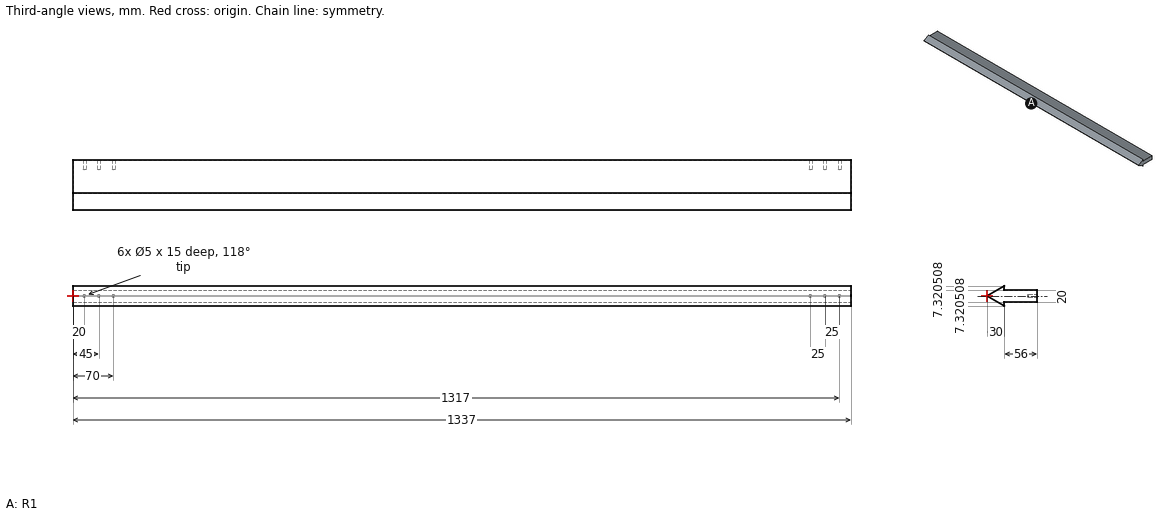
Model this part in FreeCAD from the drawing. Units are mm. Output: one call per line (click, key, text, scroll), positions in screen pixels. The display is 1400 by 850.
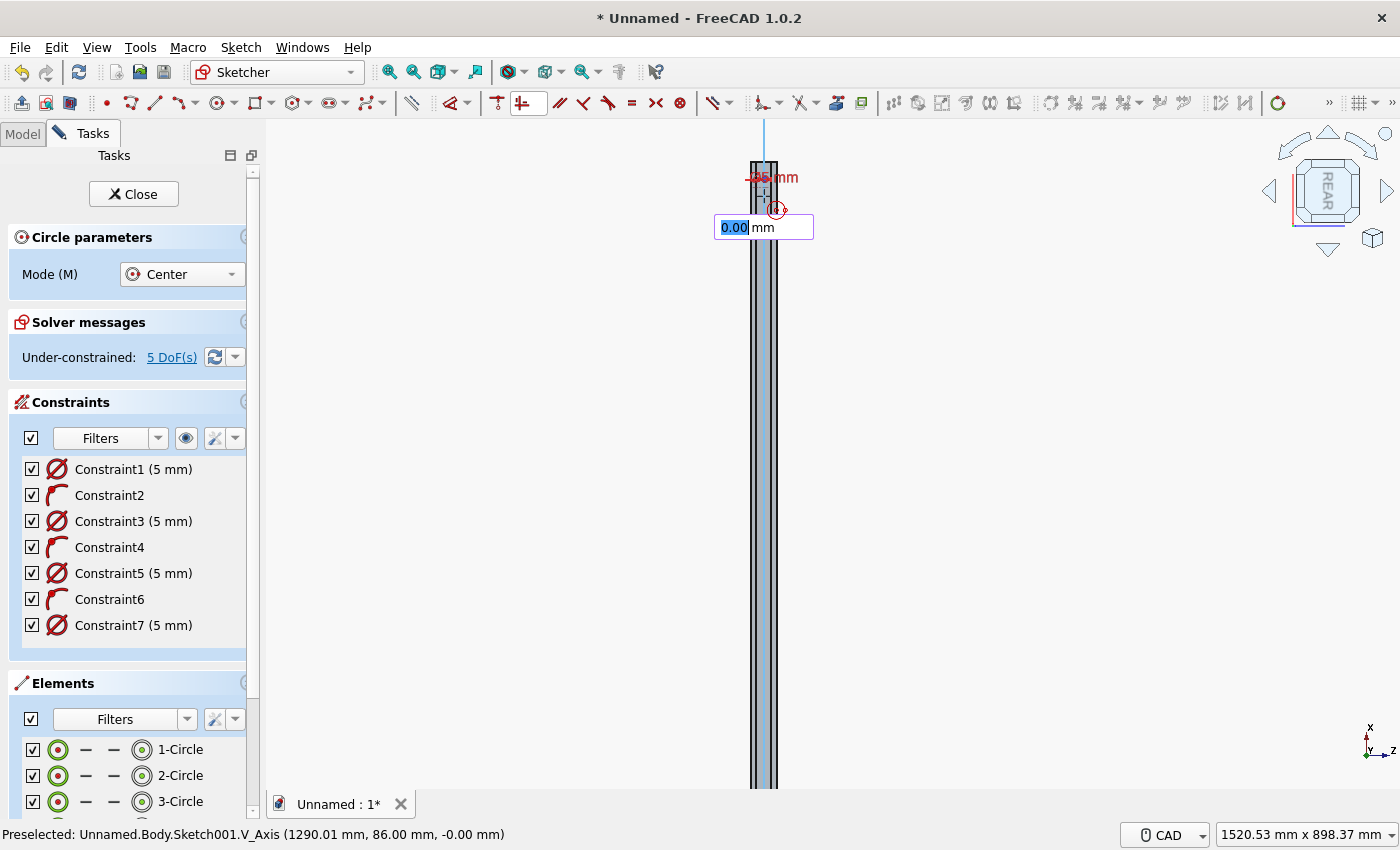
scroll(765, 195, up, 12)
move(766, 193)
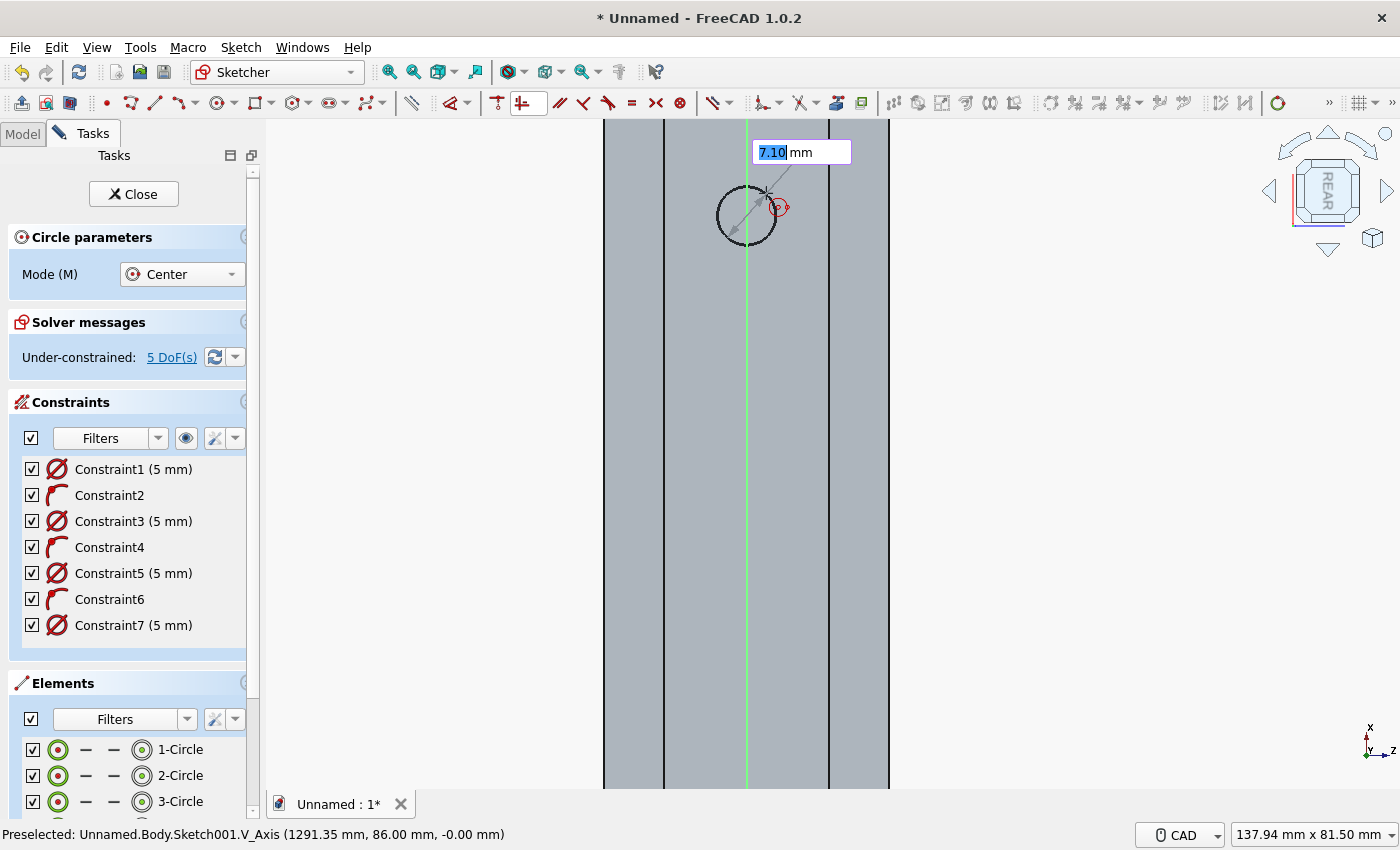
text(5)
key(Return)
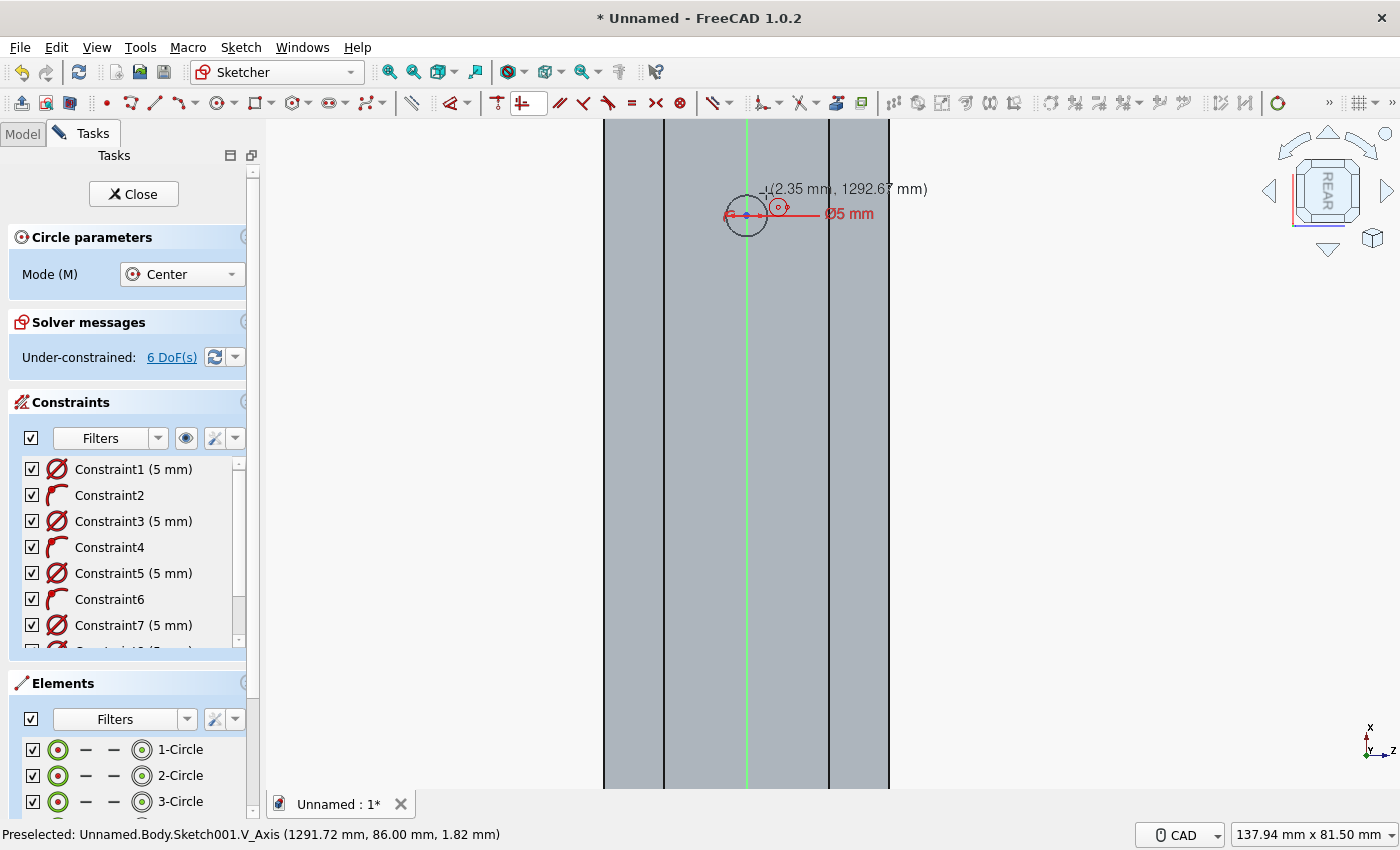
scroll(765, 195, down, 15)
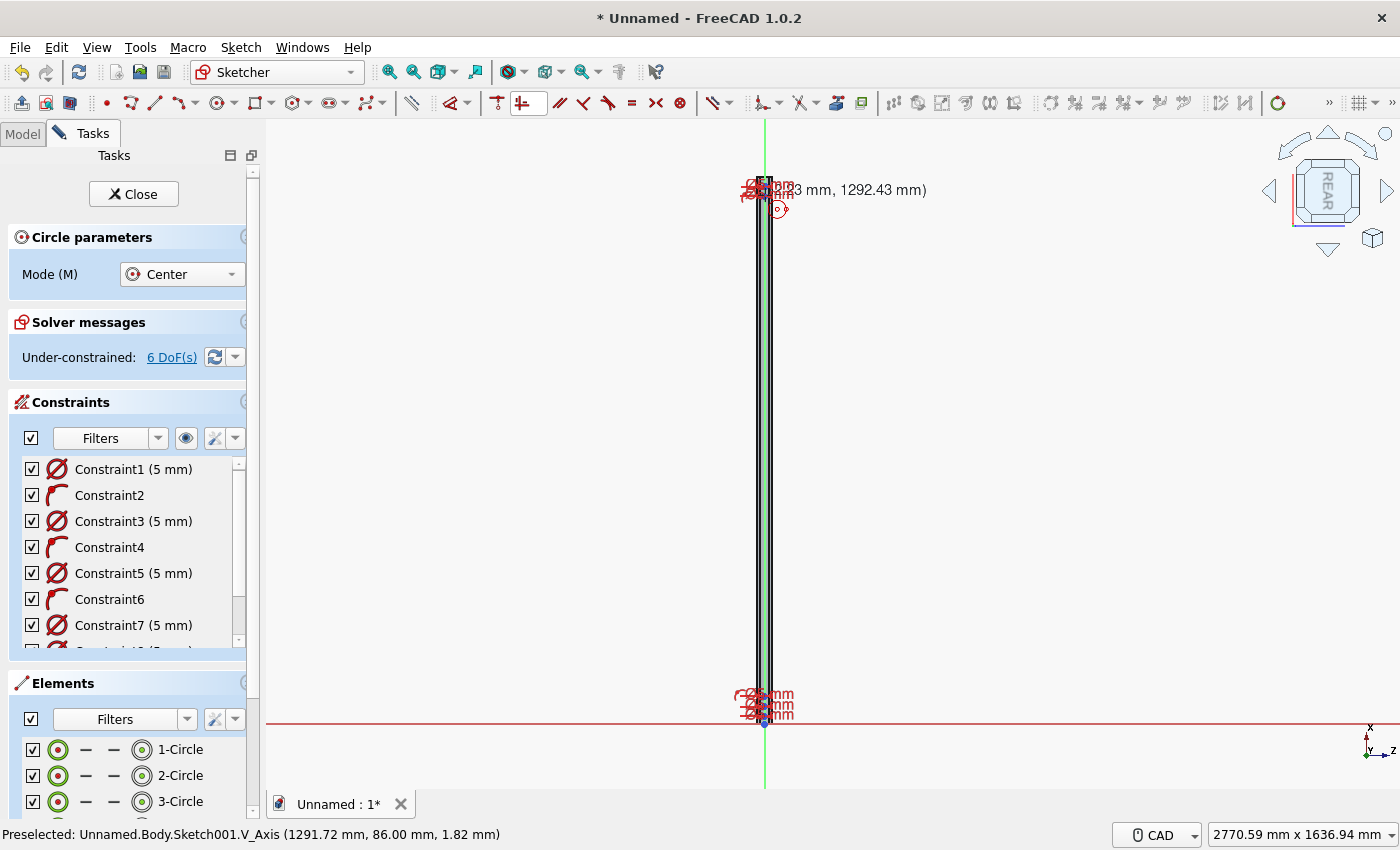
scroll(765, 206, up, 3)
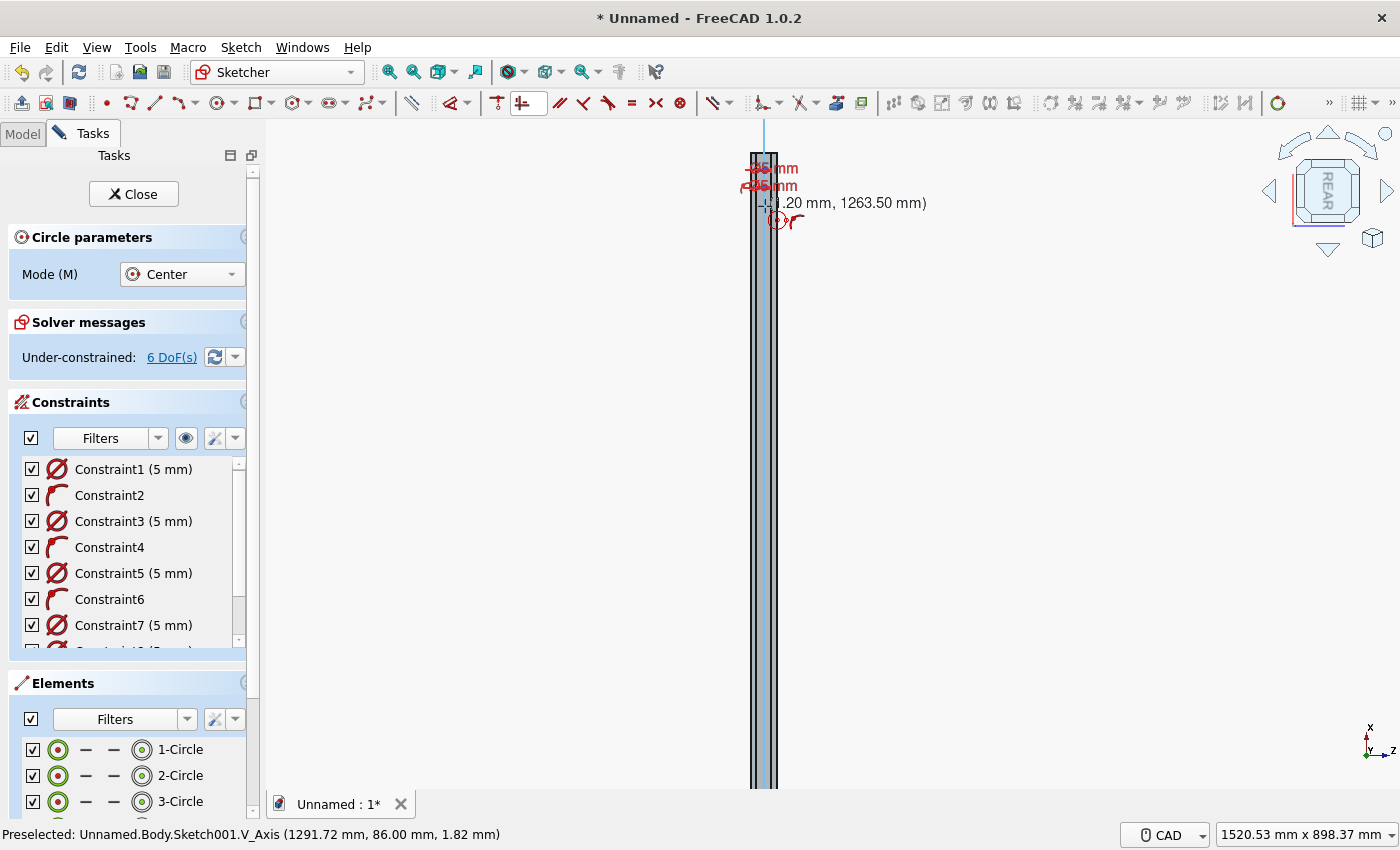
click(764, 205)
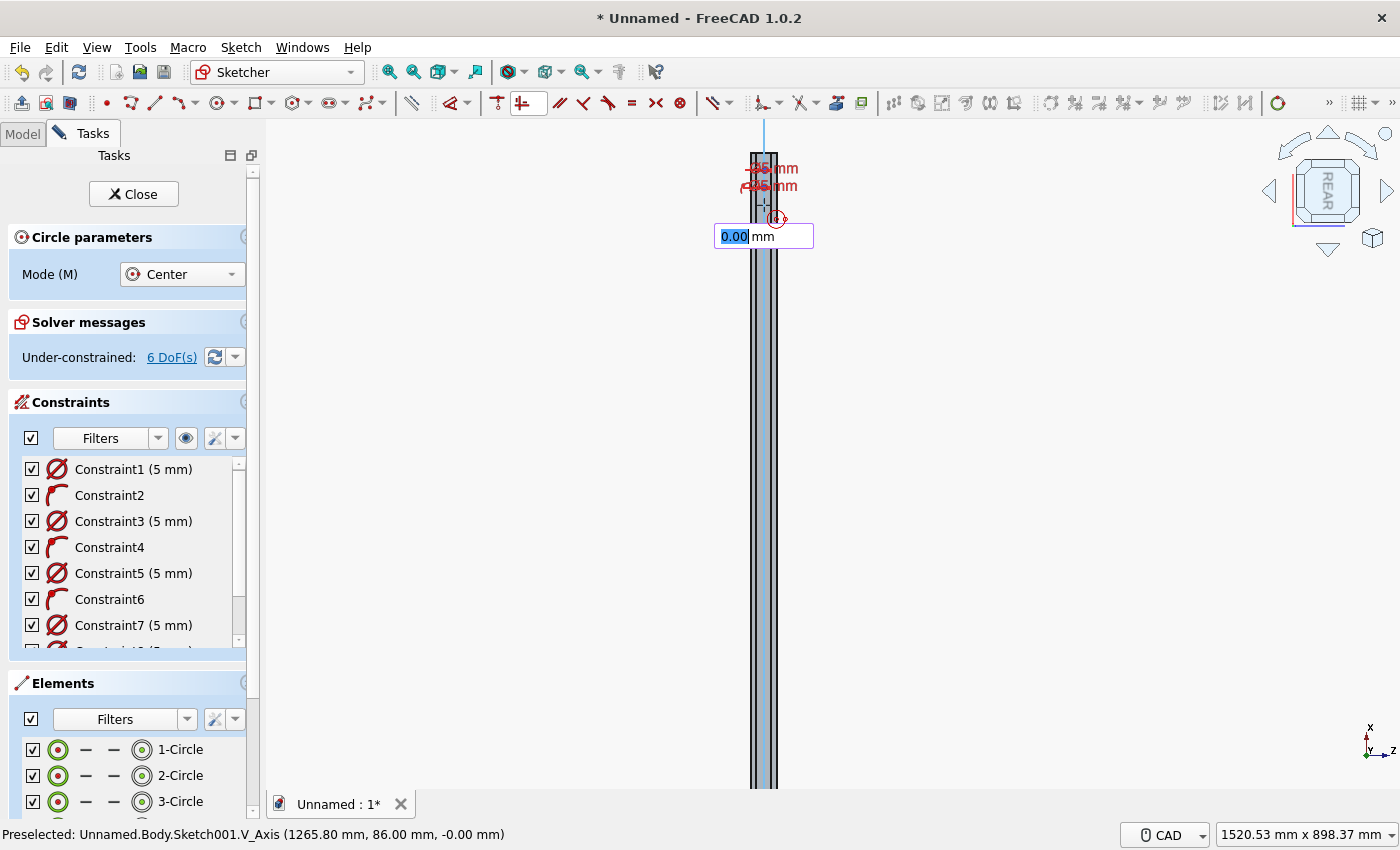
scroll(765, 204, up, 12)
move(766, 208)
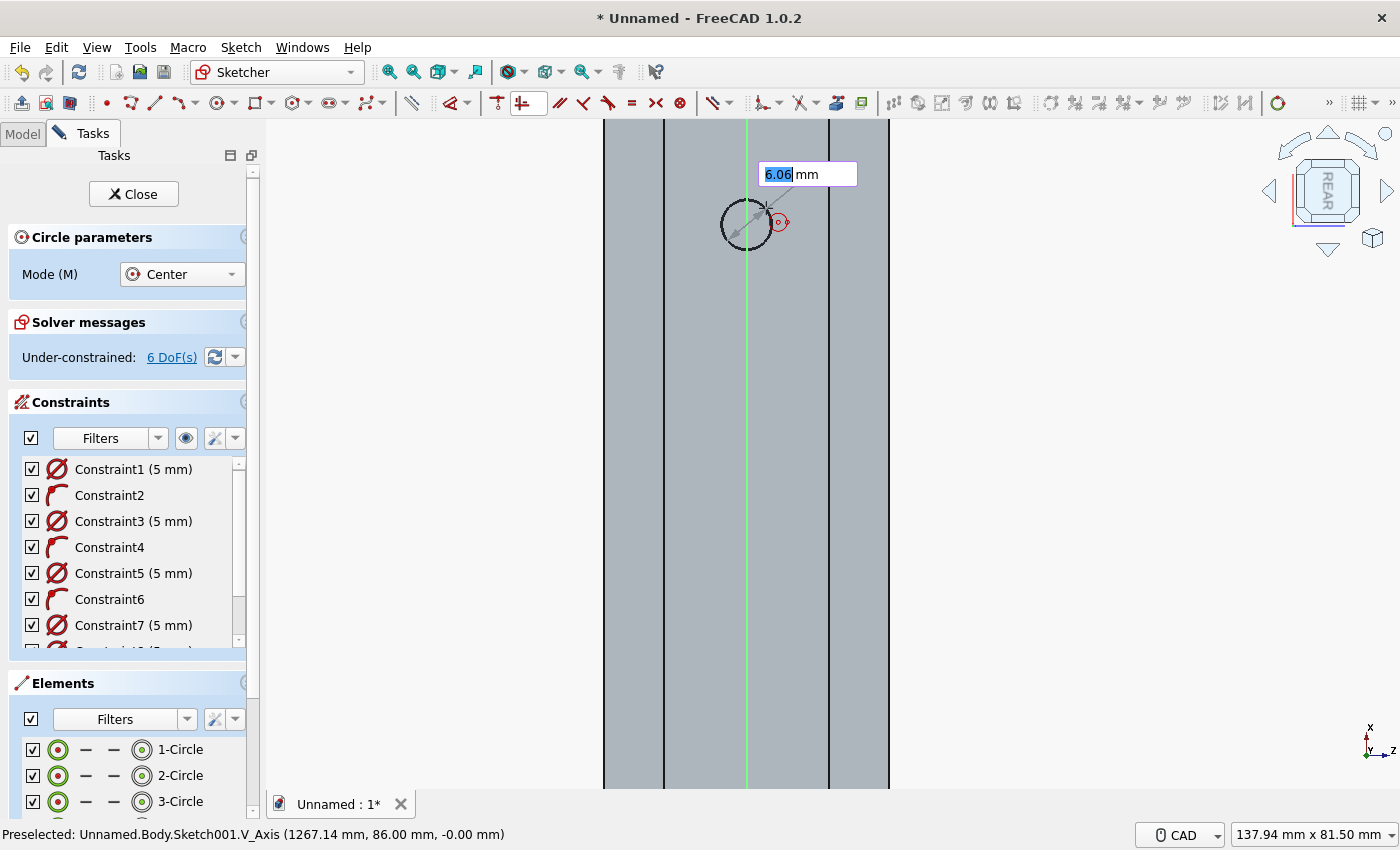
text(5)
key(Return)
key(Escape)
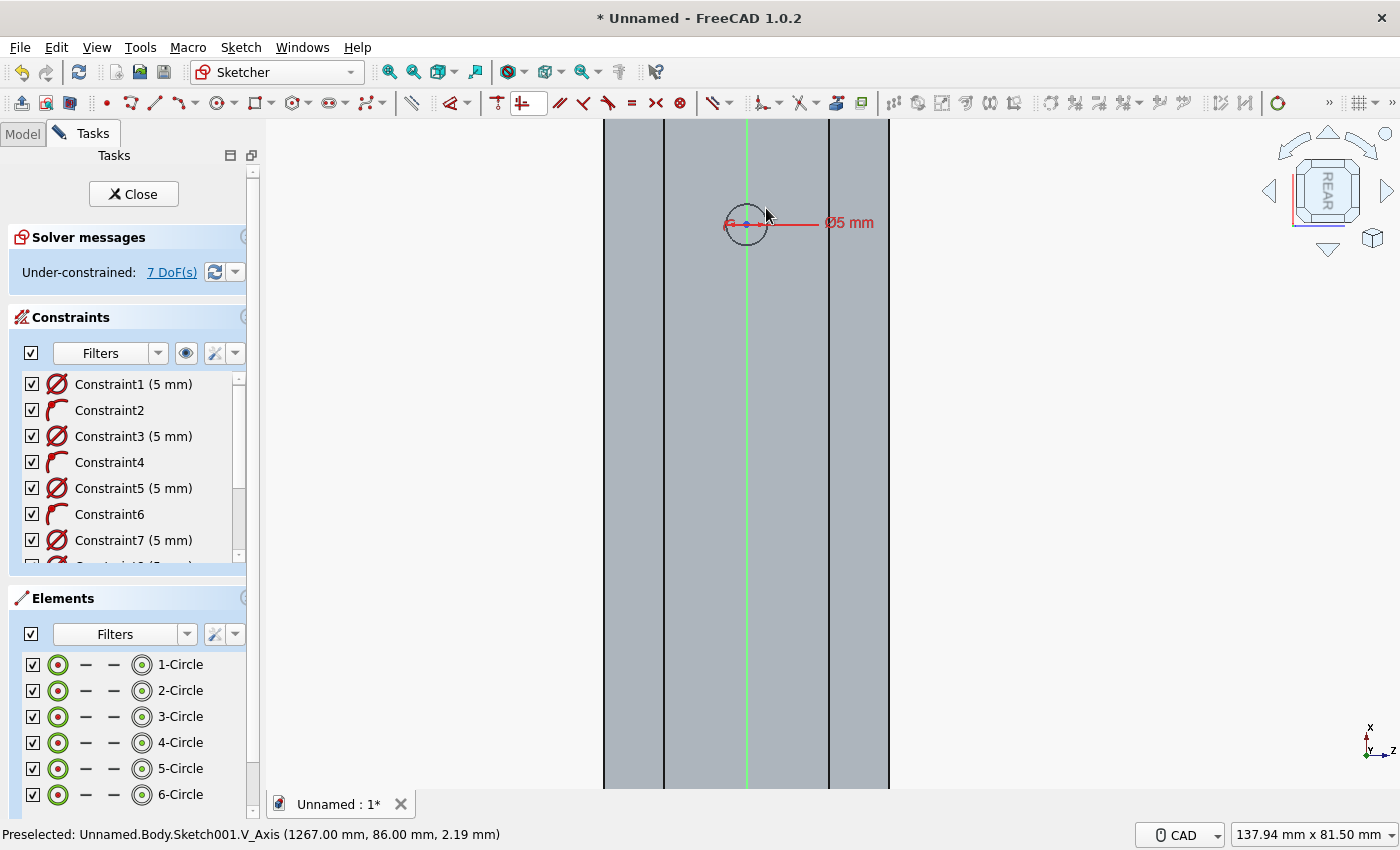
scroll(765, 205, down, 15)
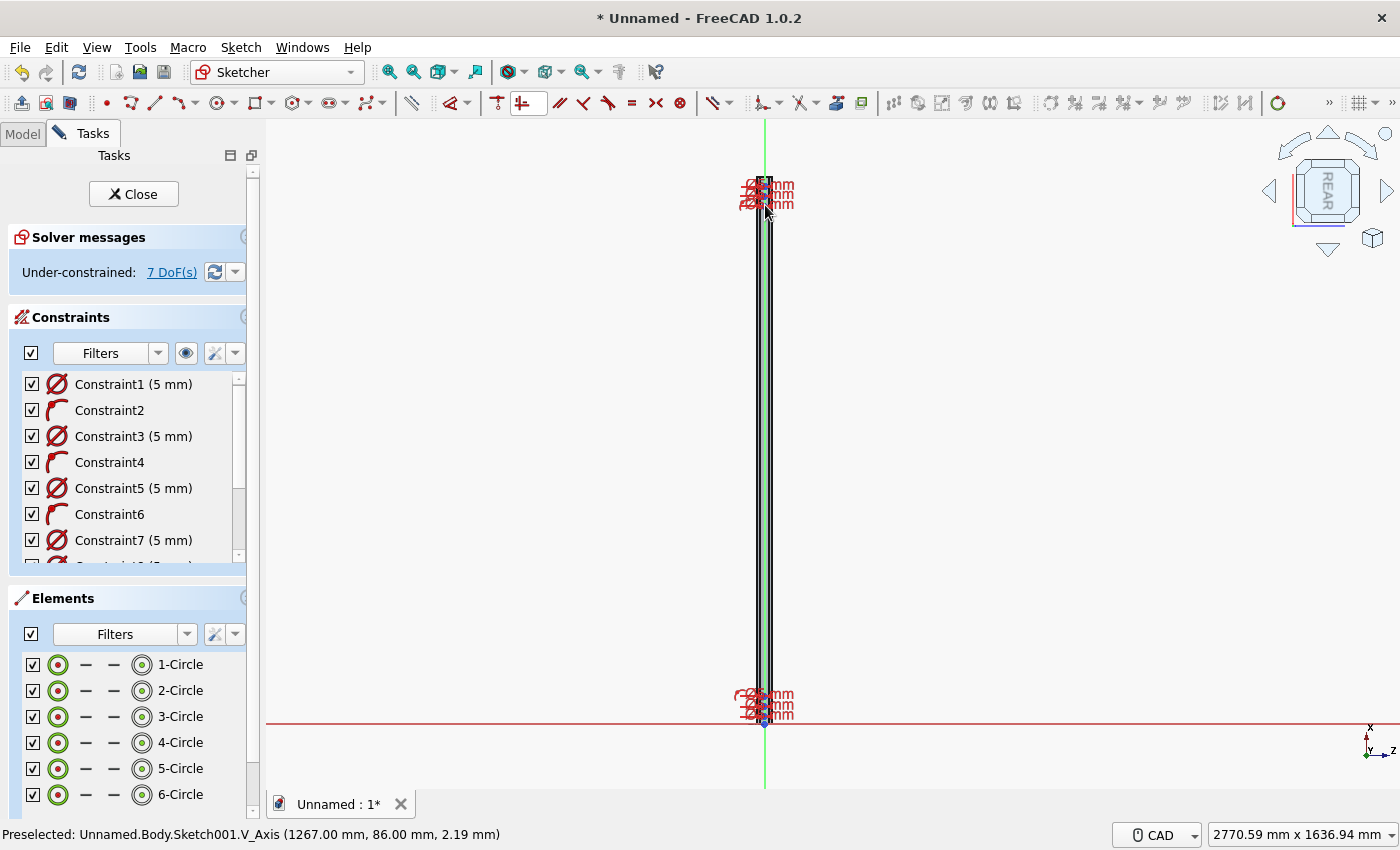
scroll(765, 187, up, 2)